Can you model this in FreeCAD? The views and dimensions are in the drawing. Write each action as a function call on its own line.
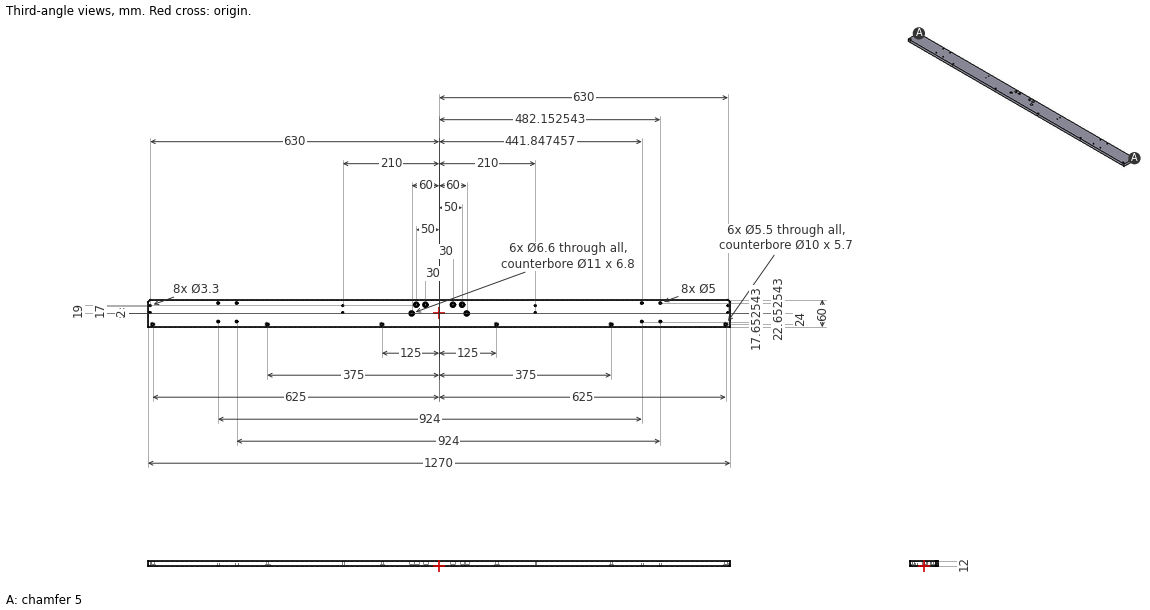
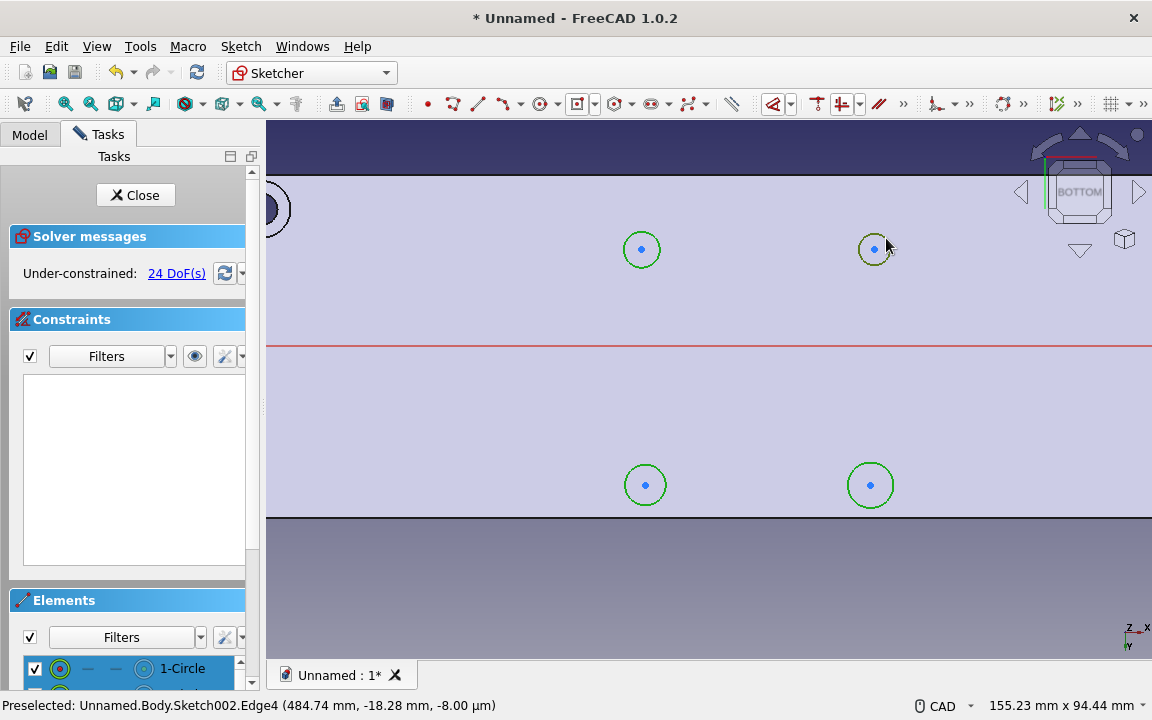
scroll(892, 392, down, 12)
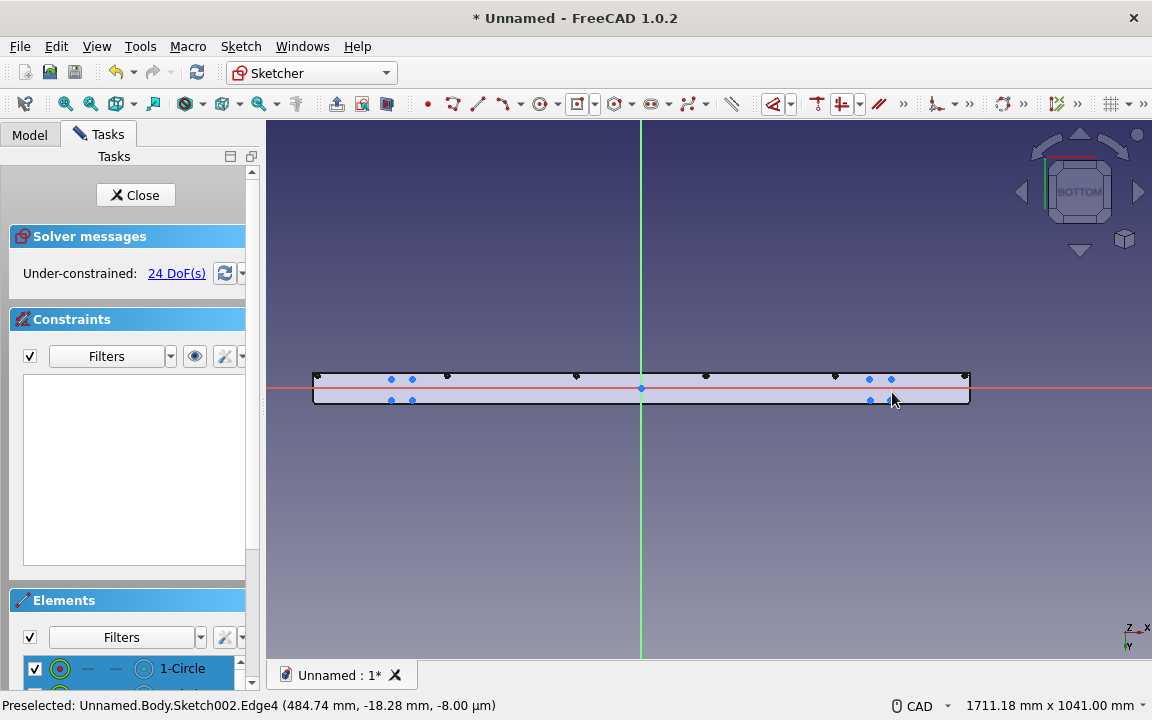
scroll(393, 379, up, 12)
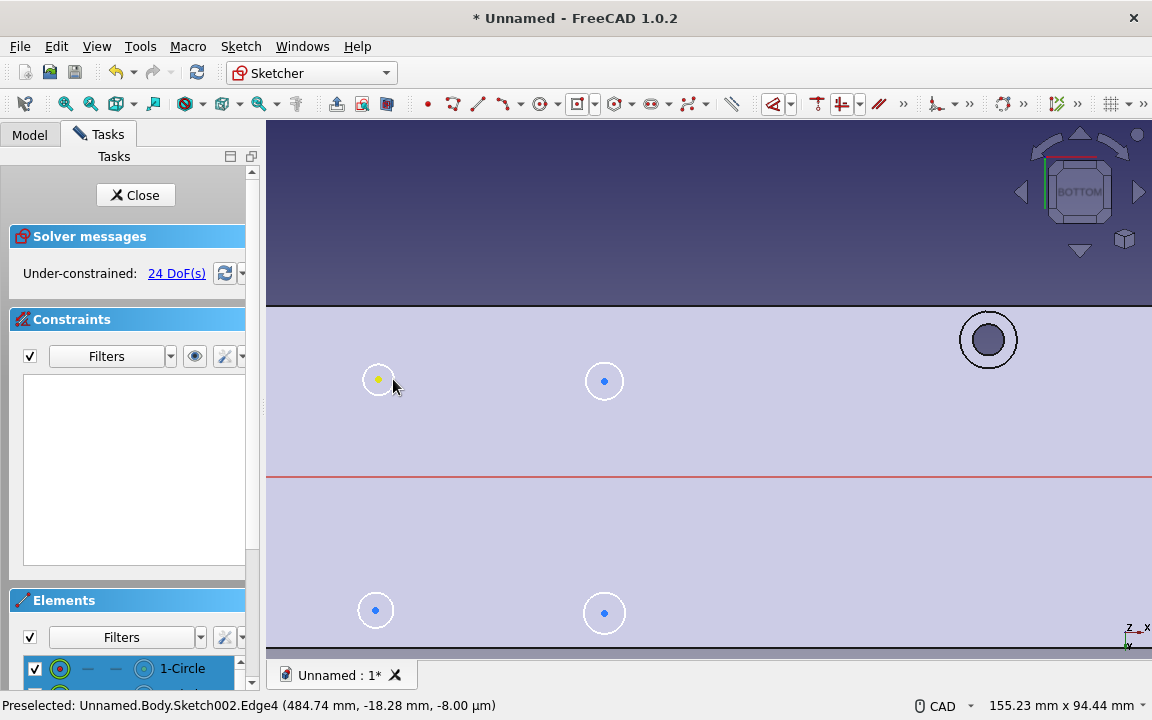
click(389, 369)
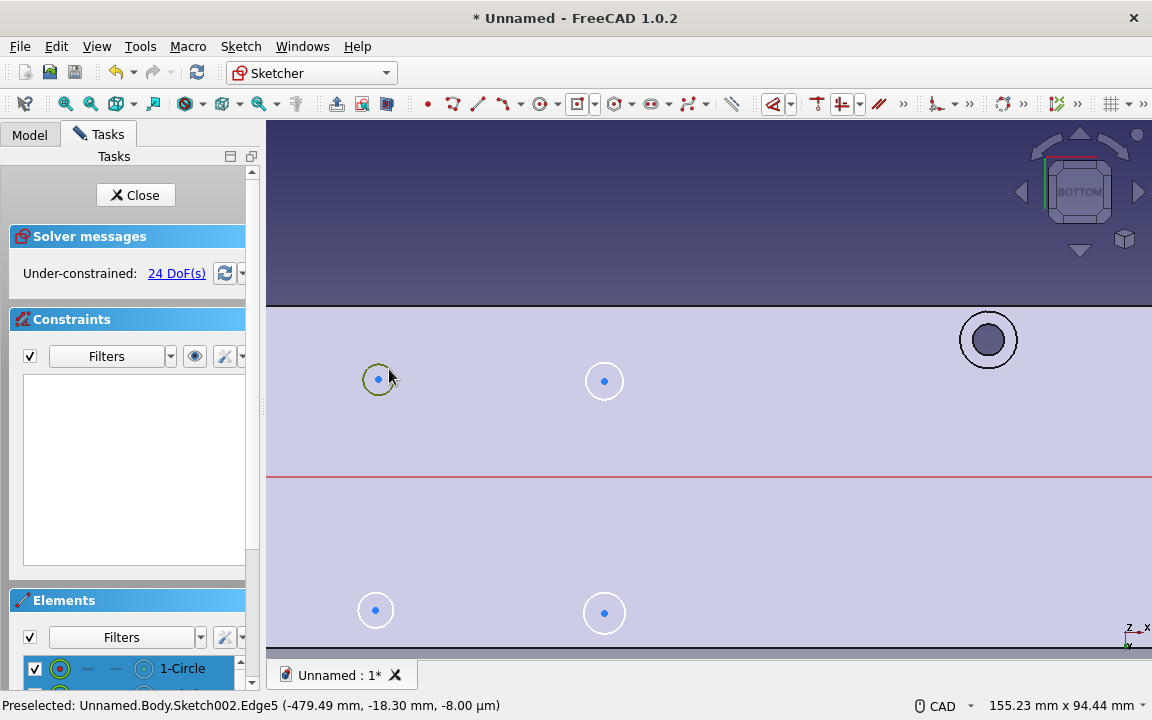
click(618, 368)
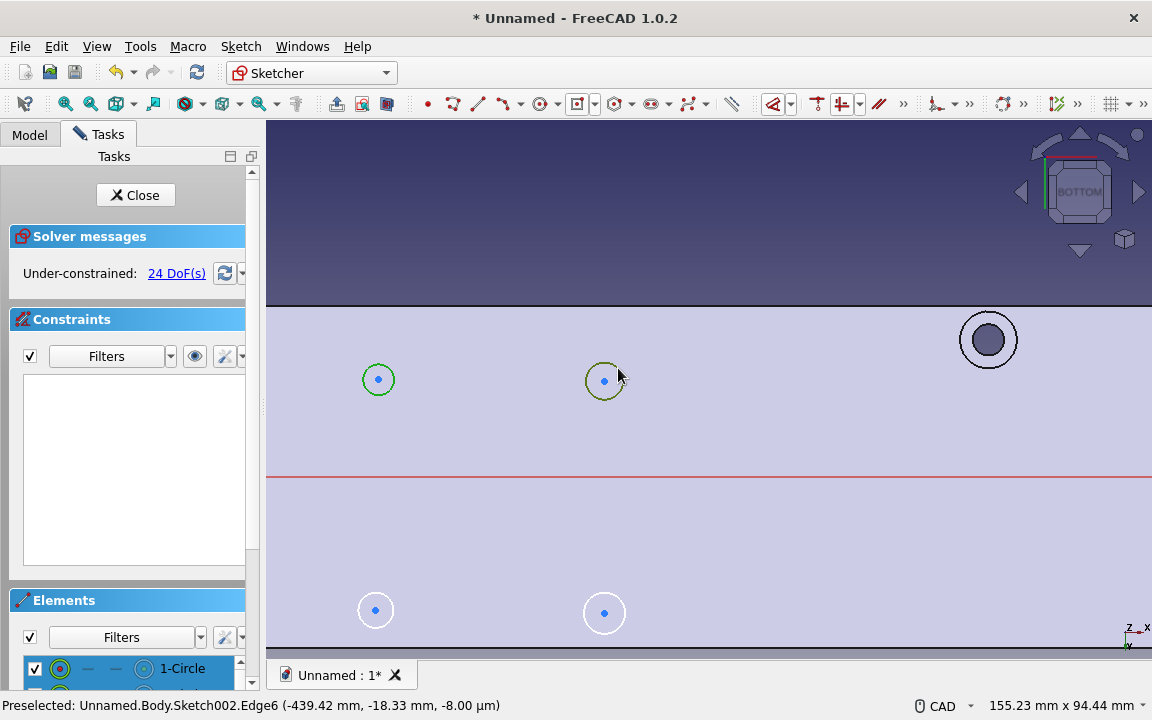
click(619, 599)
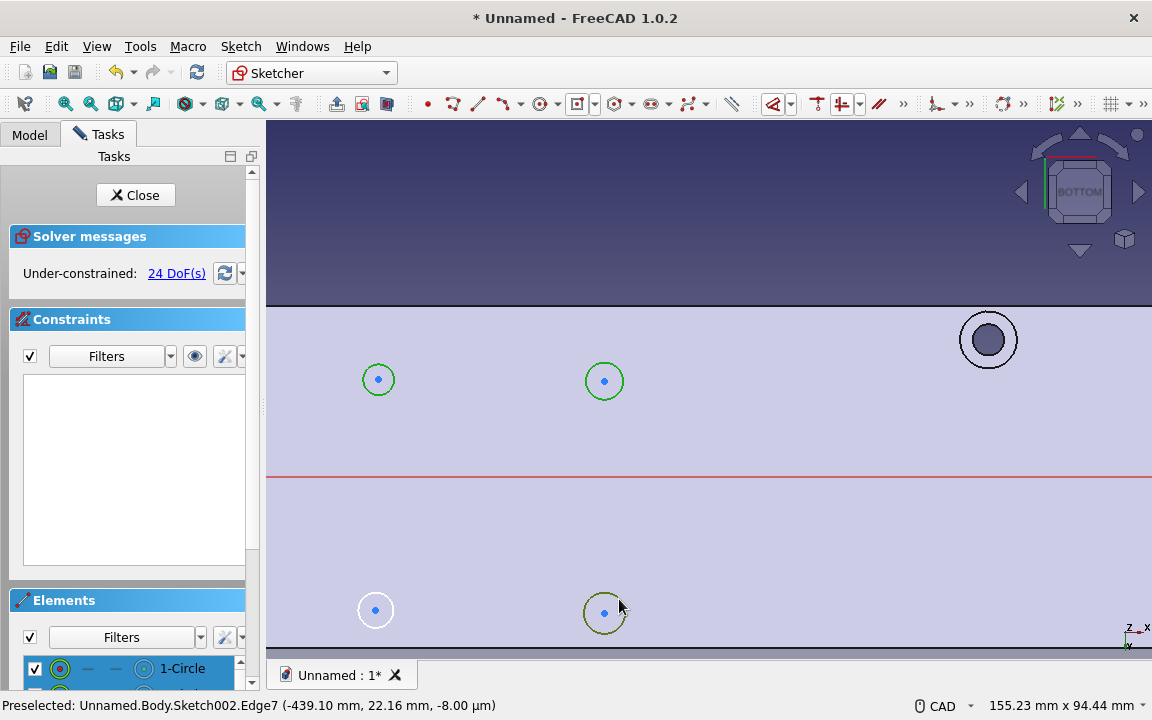
click(388, 598)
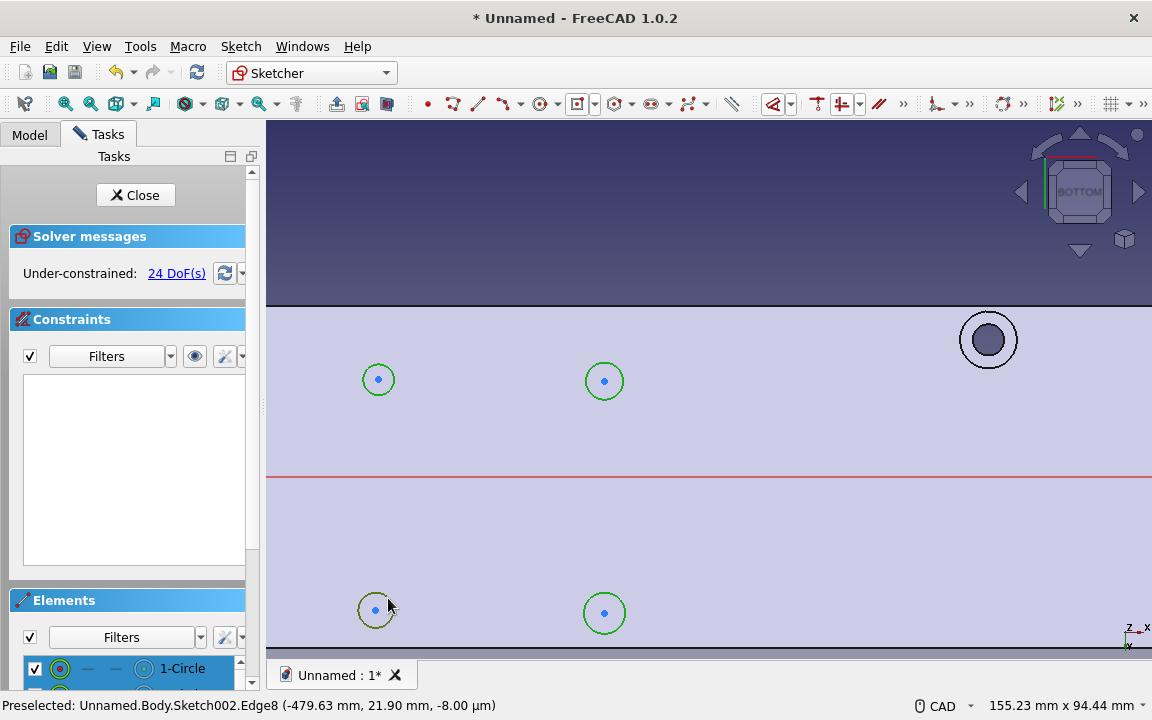
key(e)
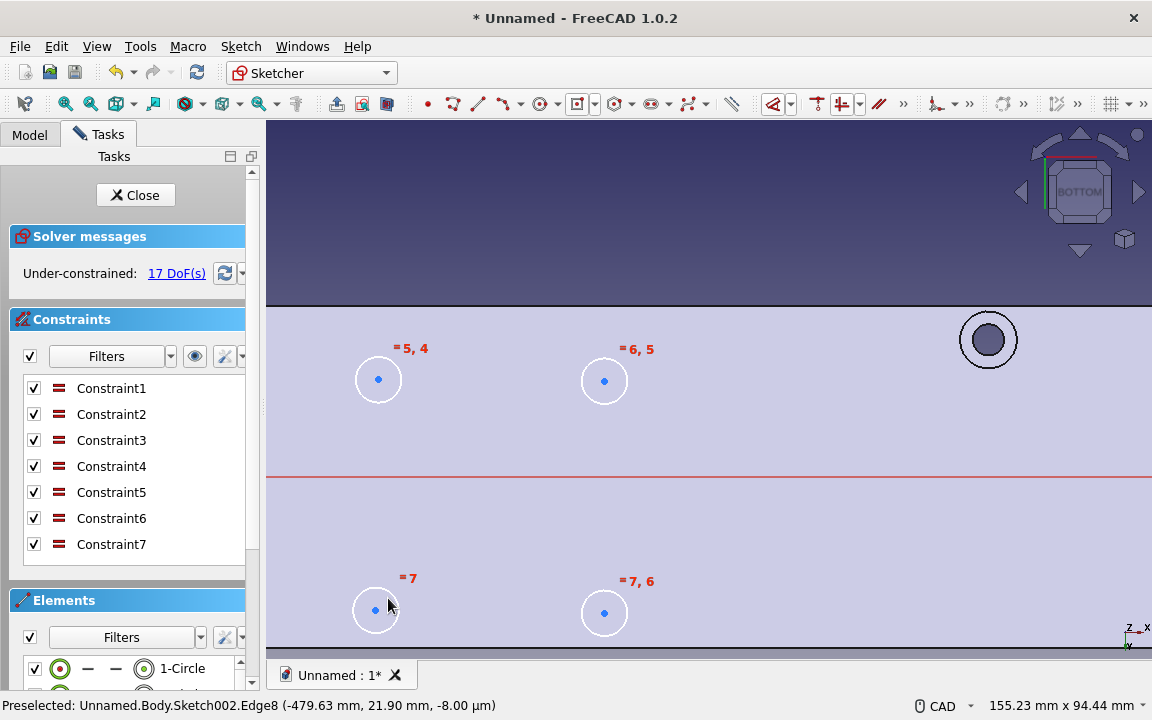
scroll(392, 379, down, 12)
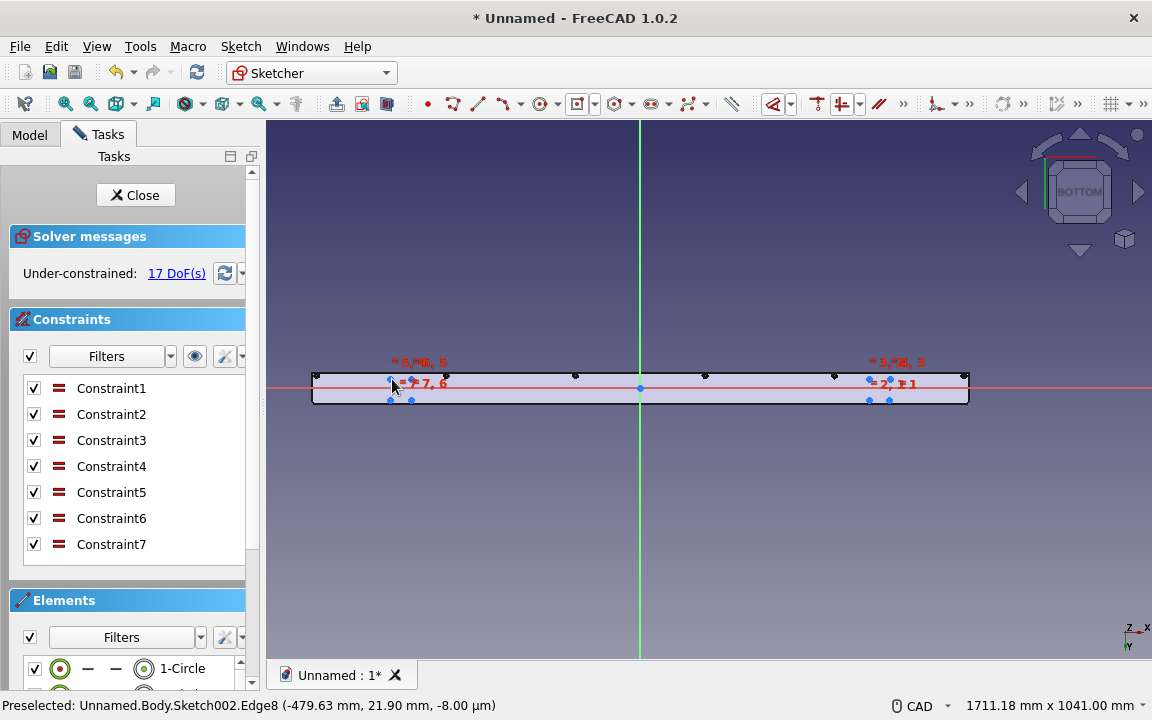
click(890, 401)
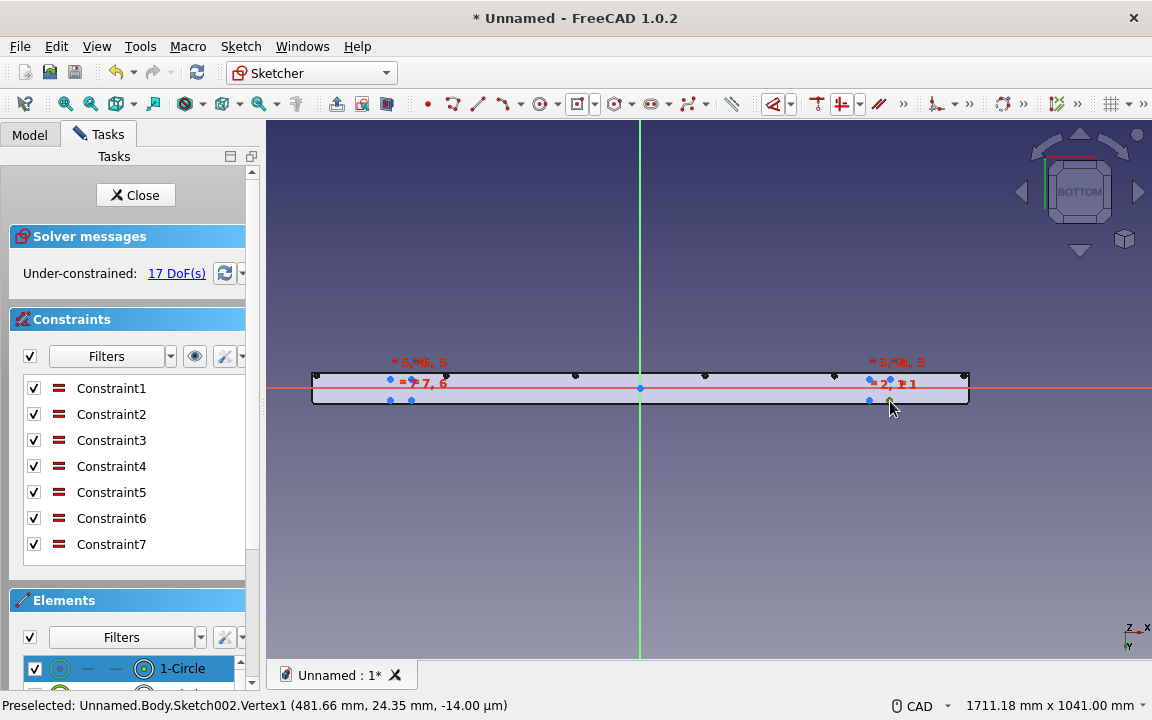
click(869, 401)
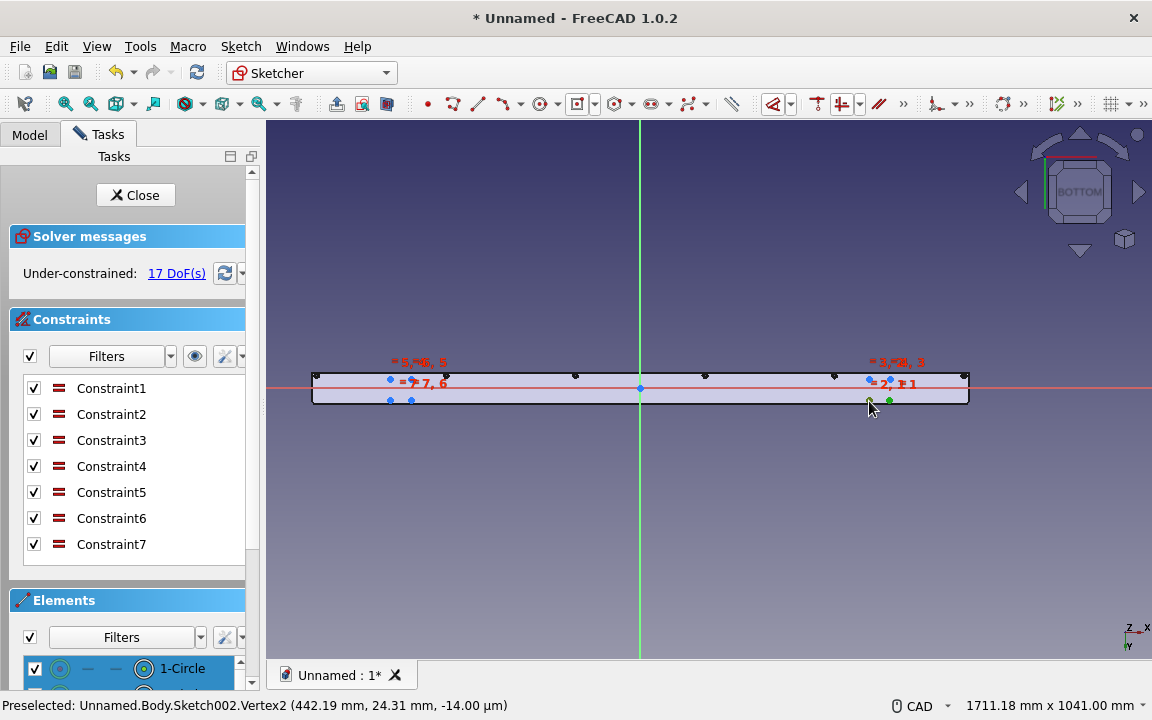
click(860, 104)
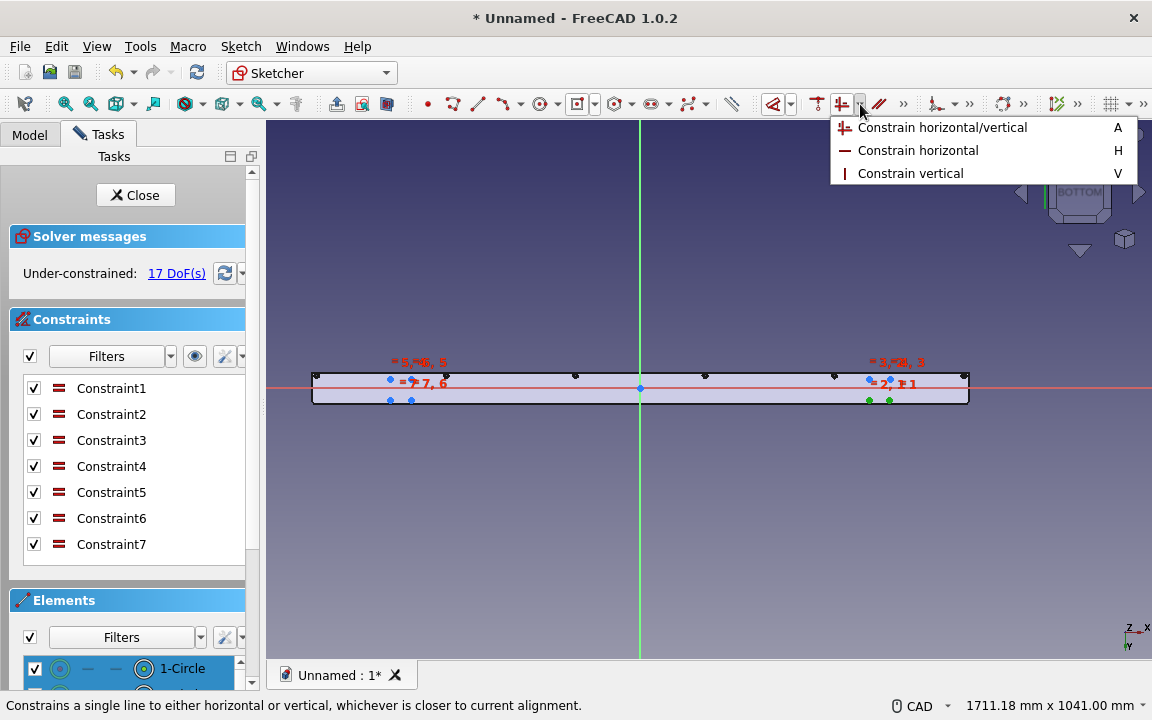
click(984, 150)